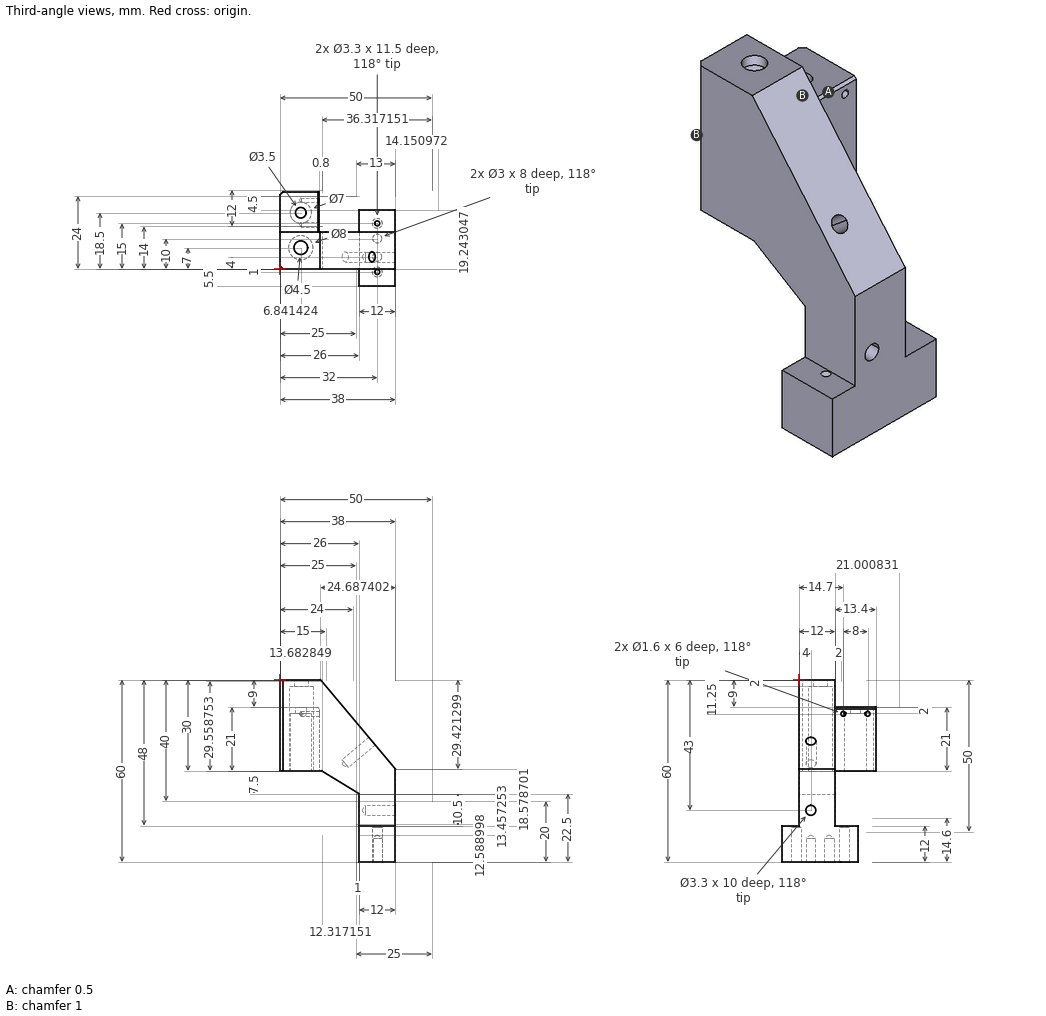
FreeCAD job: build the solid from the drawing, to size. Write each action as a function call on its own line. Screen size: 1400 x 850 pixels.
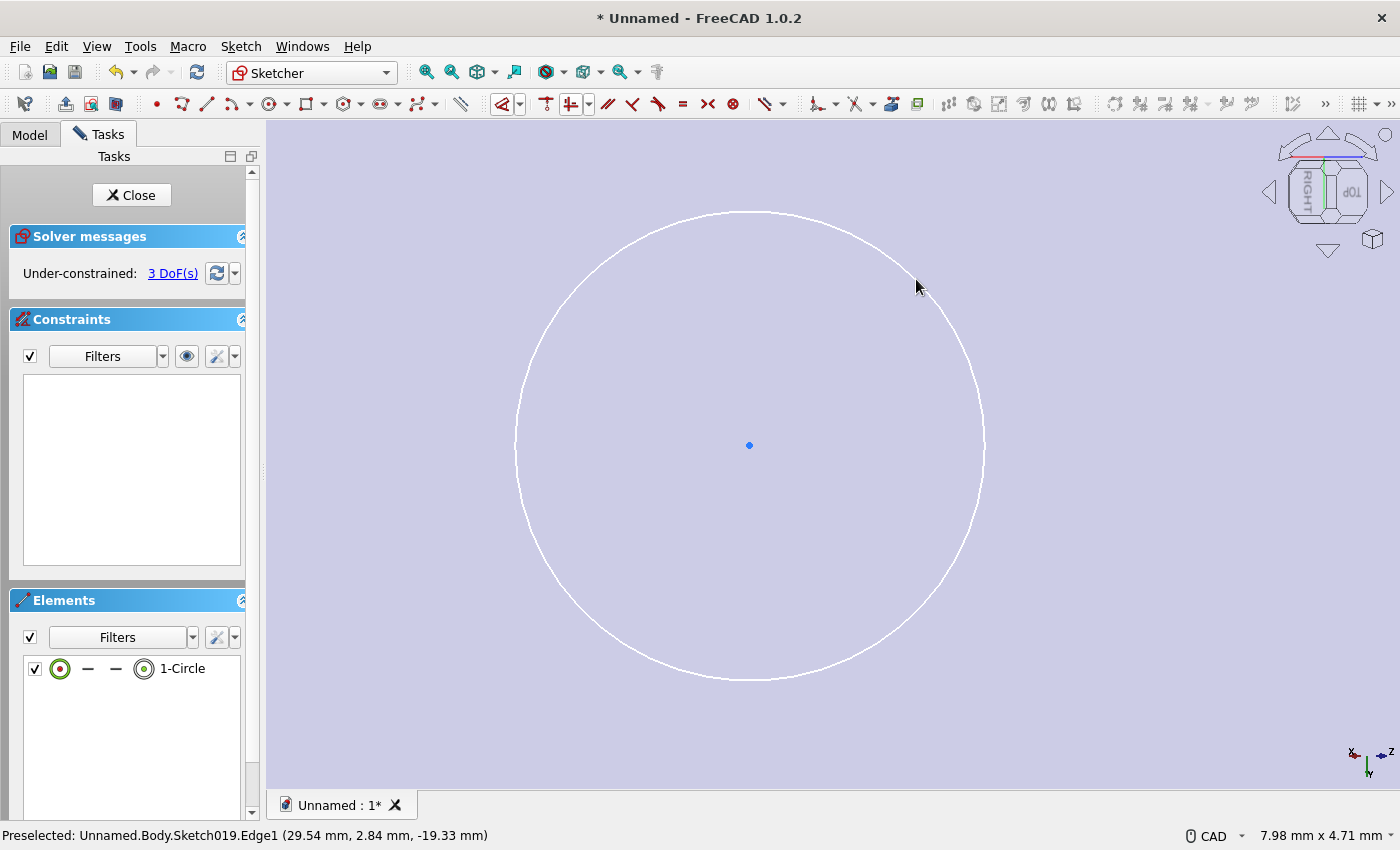
click(915, 279)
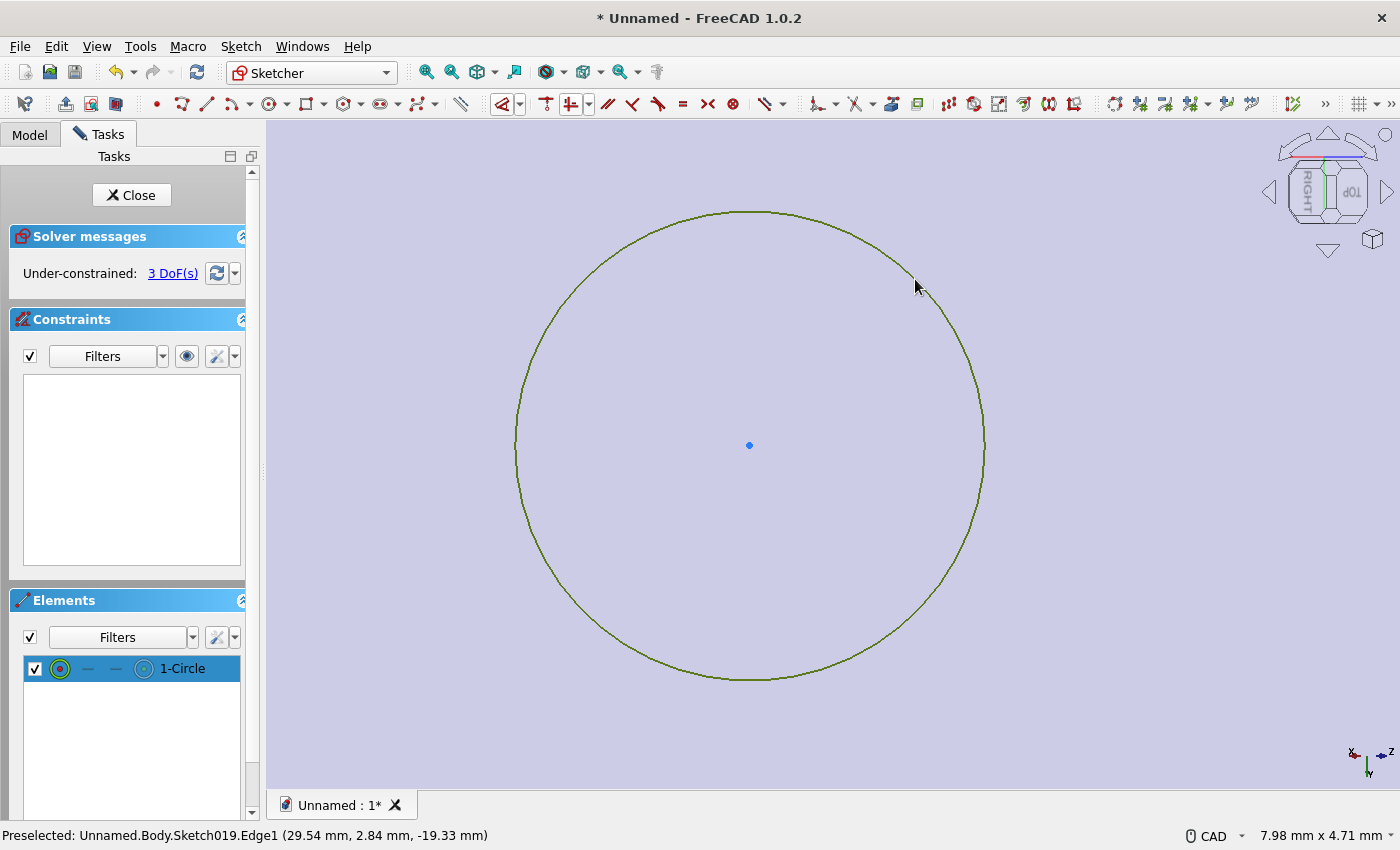
click(520, 104)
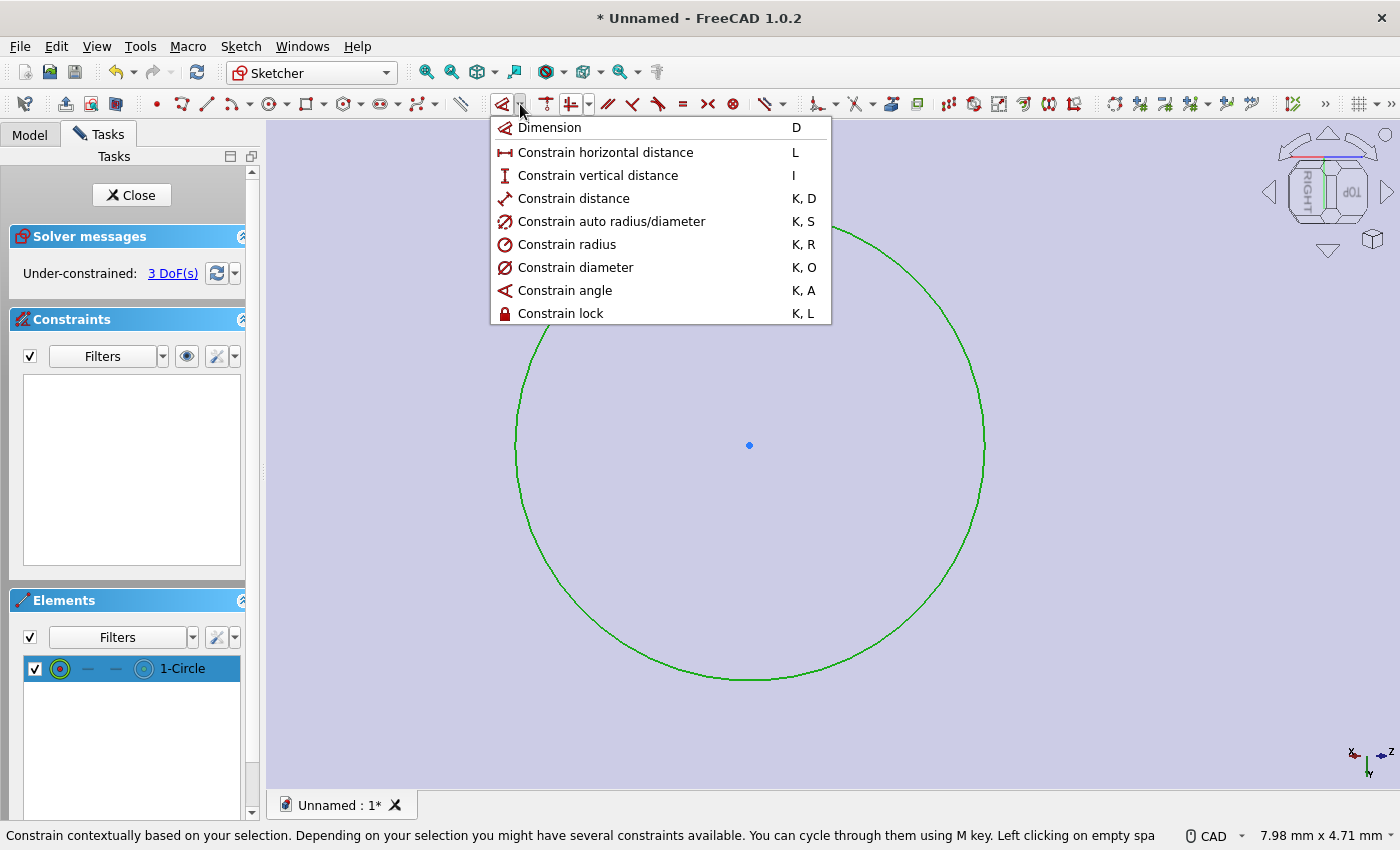
click(661, 268)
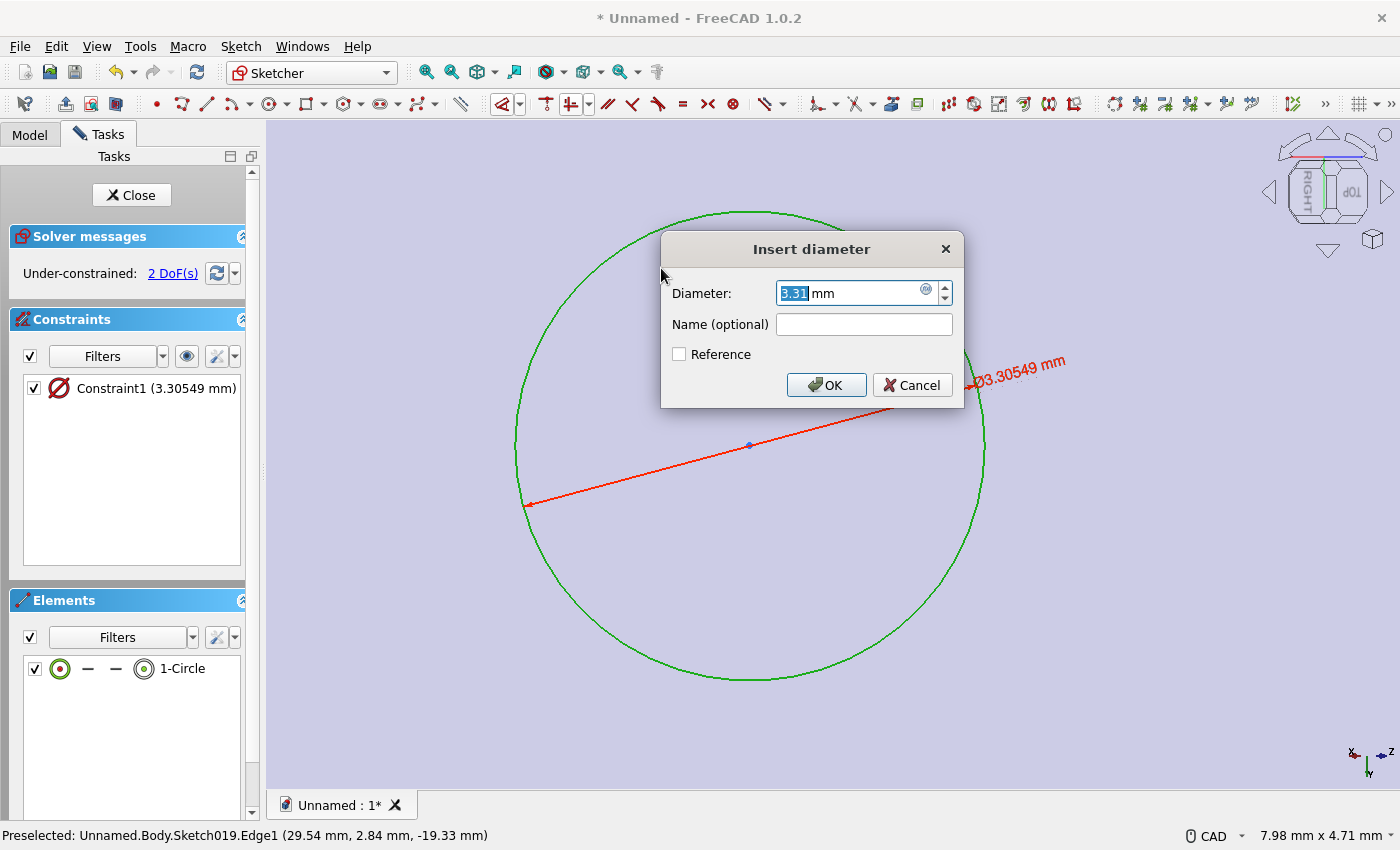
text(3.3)
key(Return)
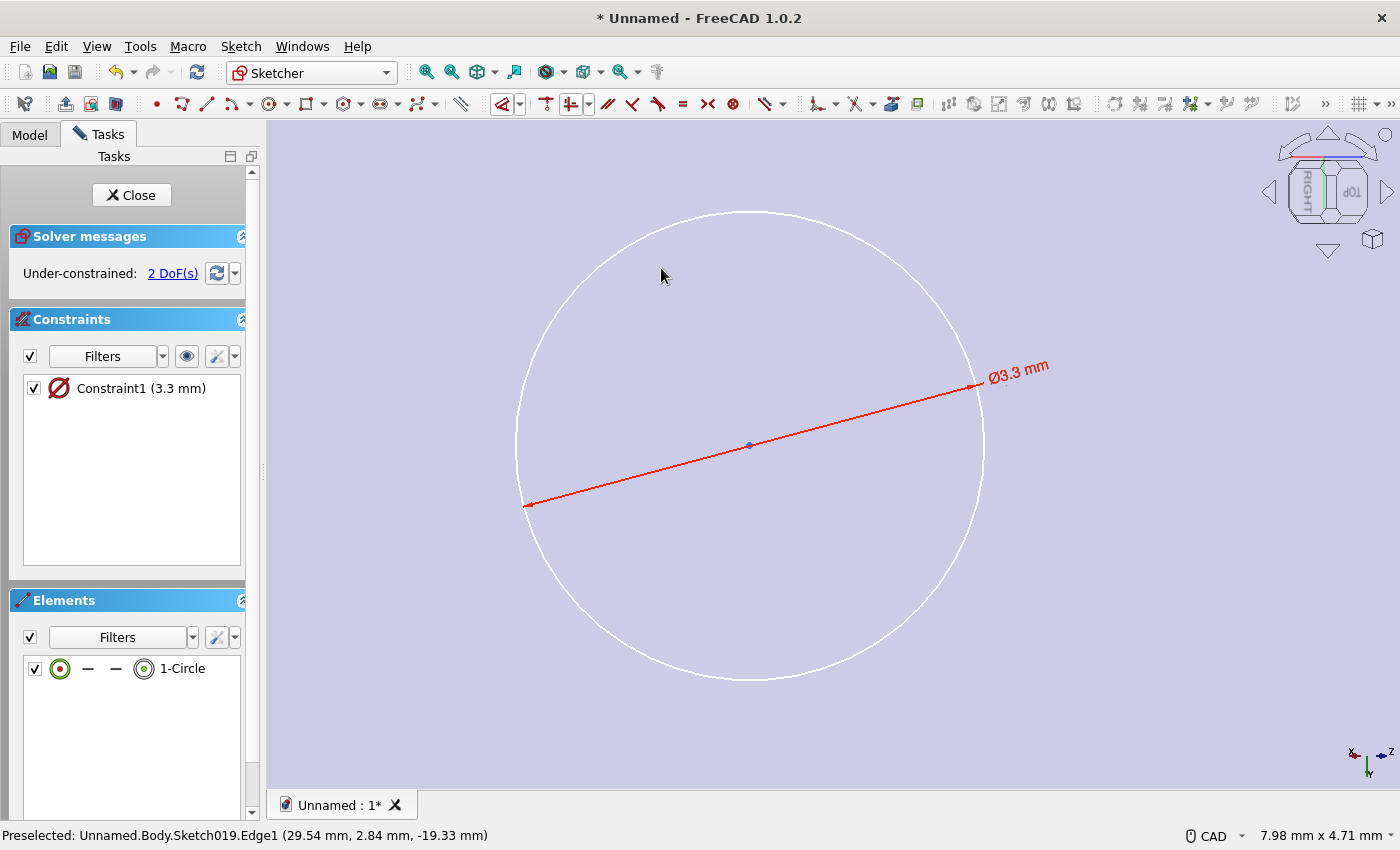
click(750, 446)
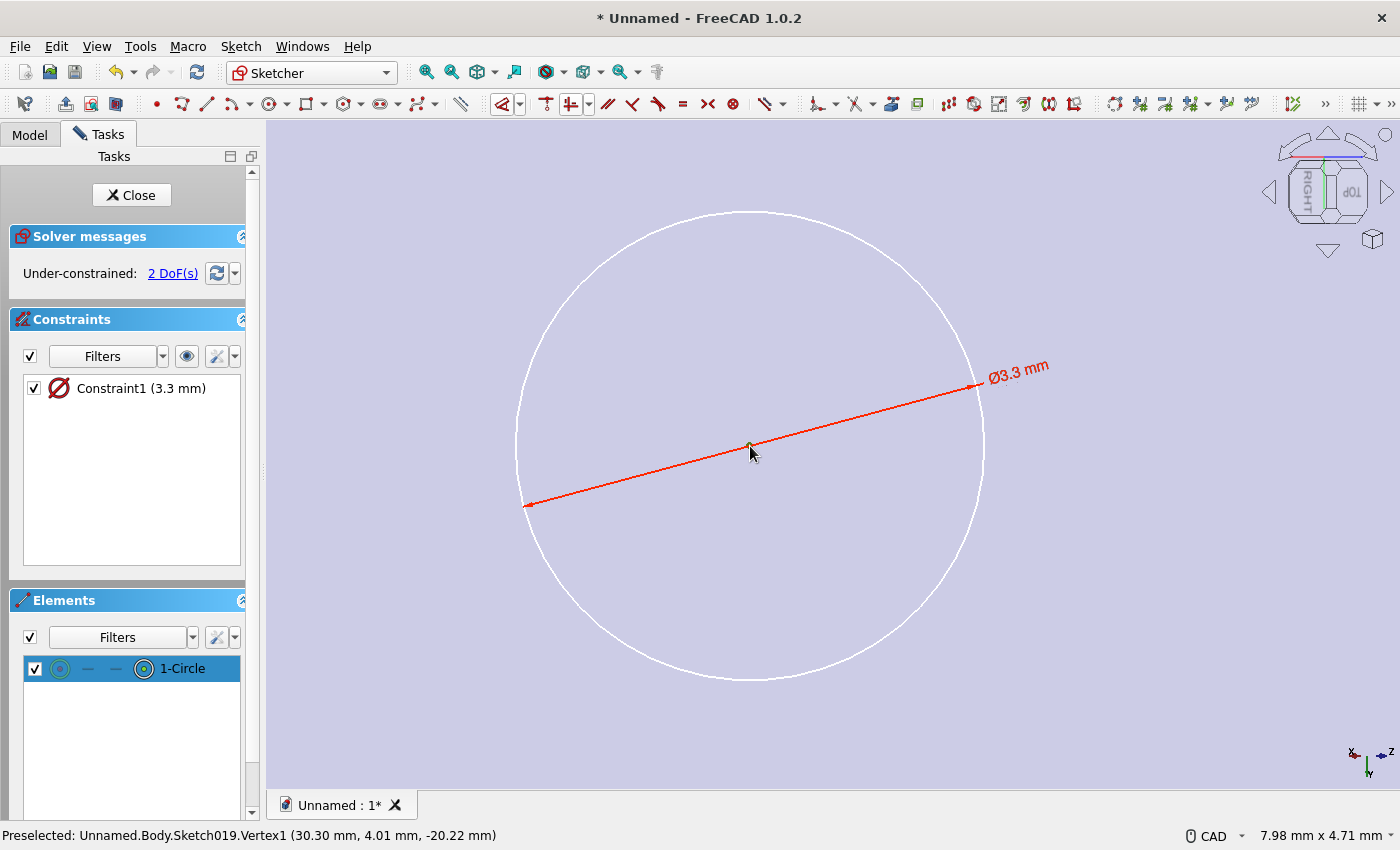
click(520, 104)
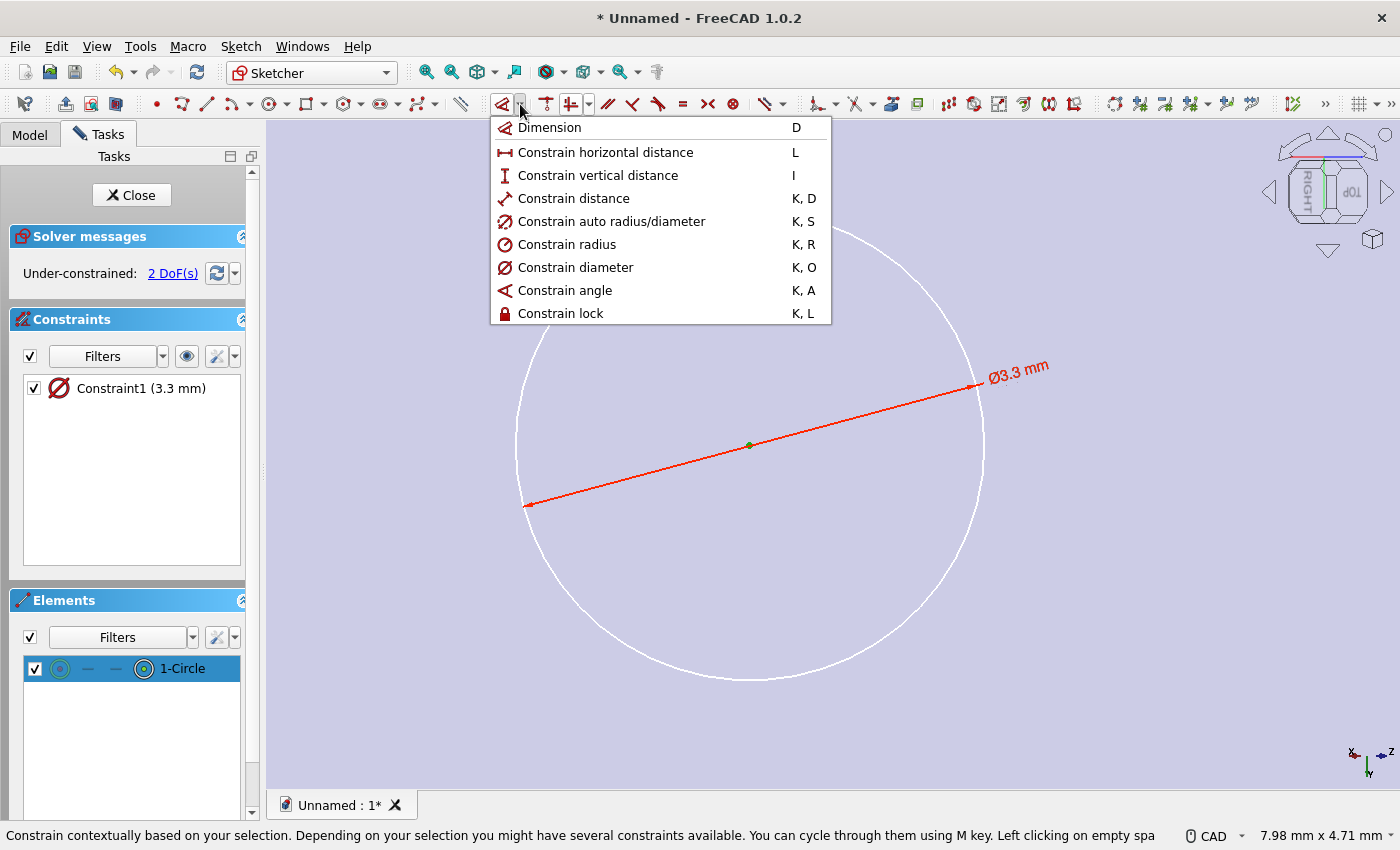
click(661, 176)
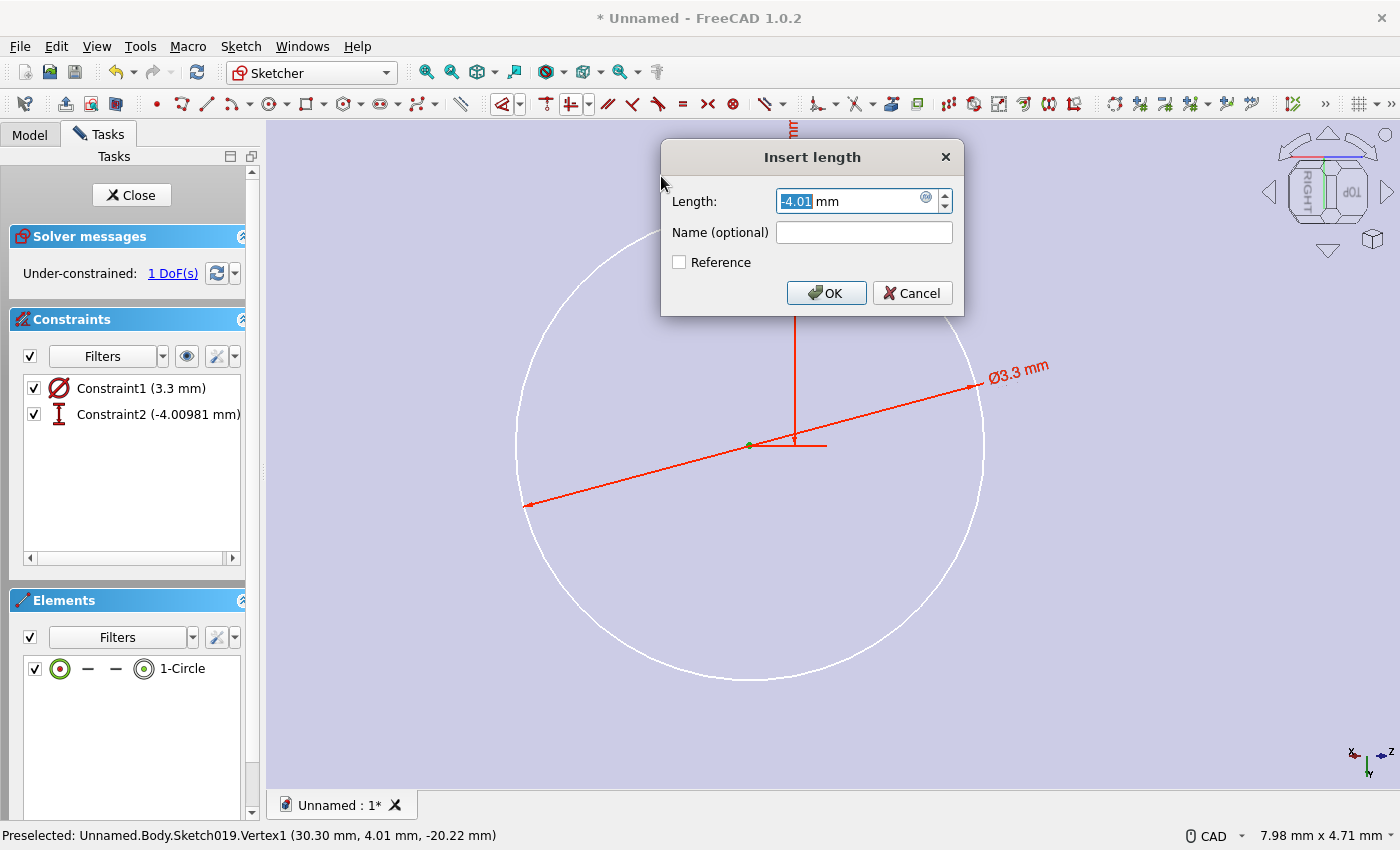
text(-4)
key(Return)